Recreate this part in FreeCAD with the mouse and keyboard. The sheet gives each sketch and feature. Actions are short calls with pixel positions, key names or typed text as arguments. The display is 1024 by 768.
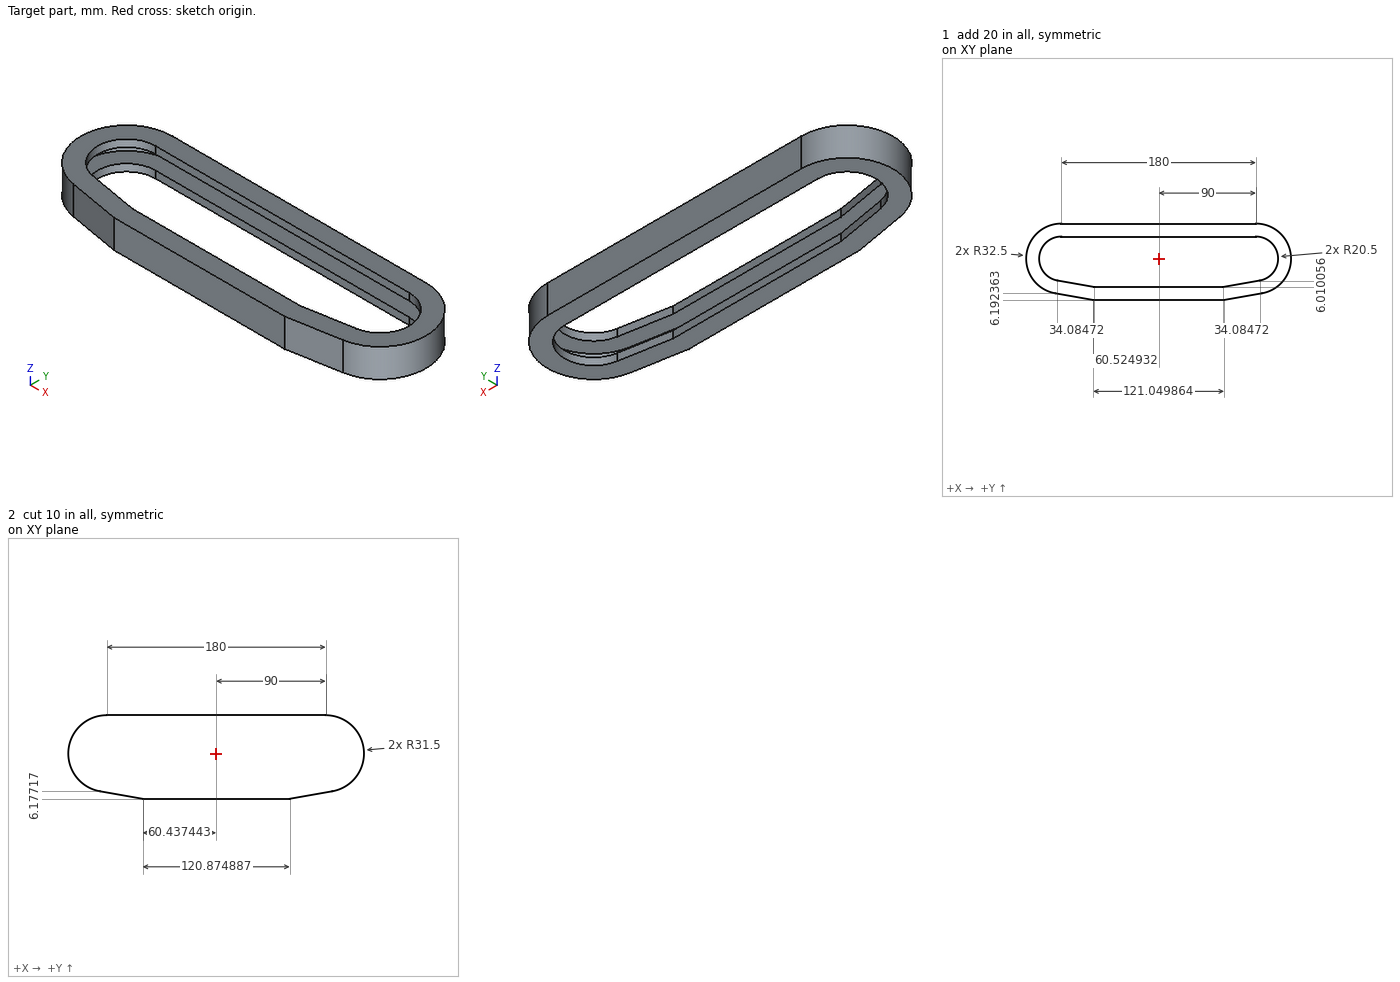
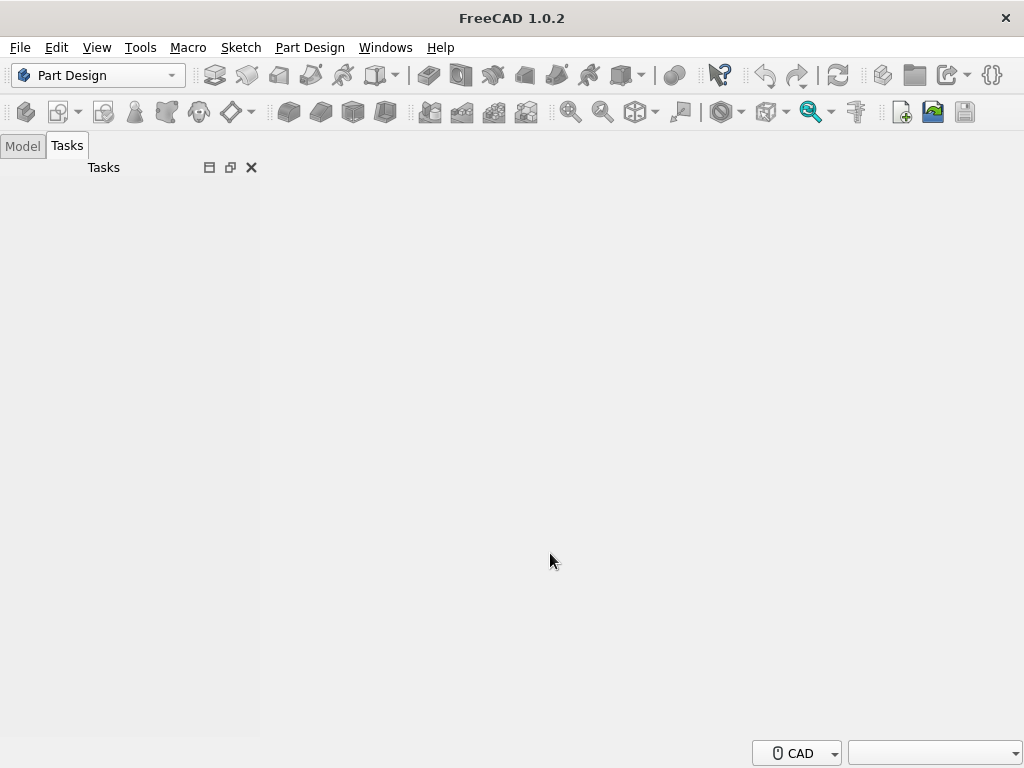
key(ctrl+n)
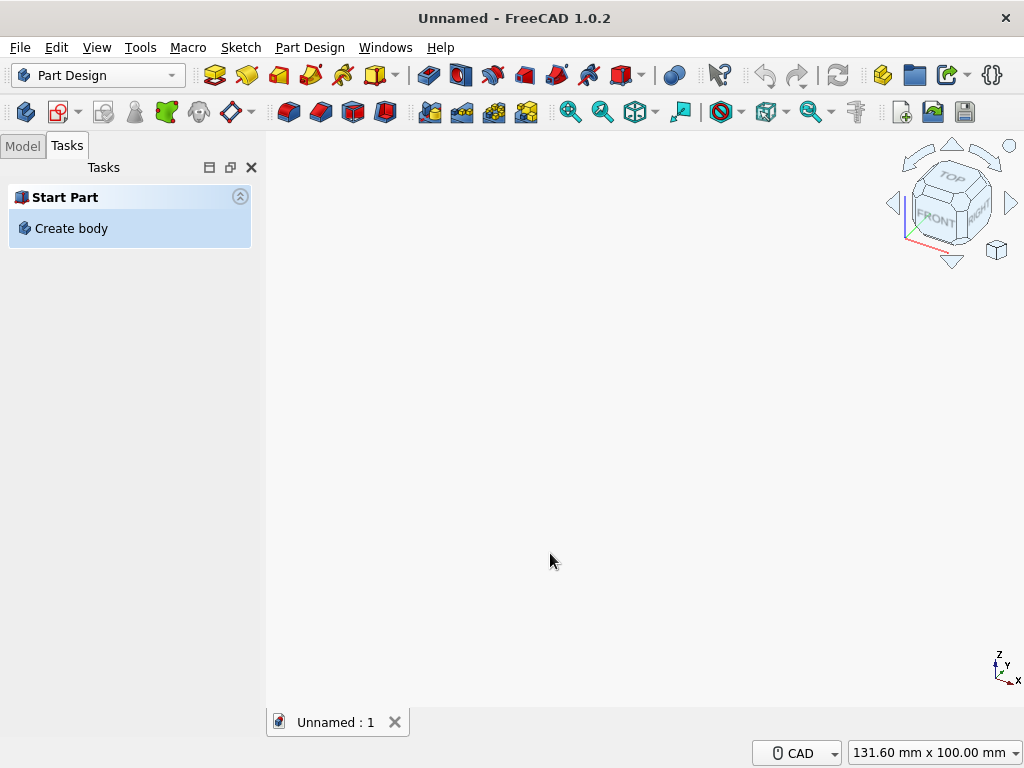
click(58, 112)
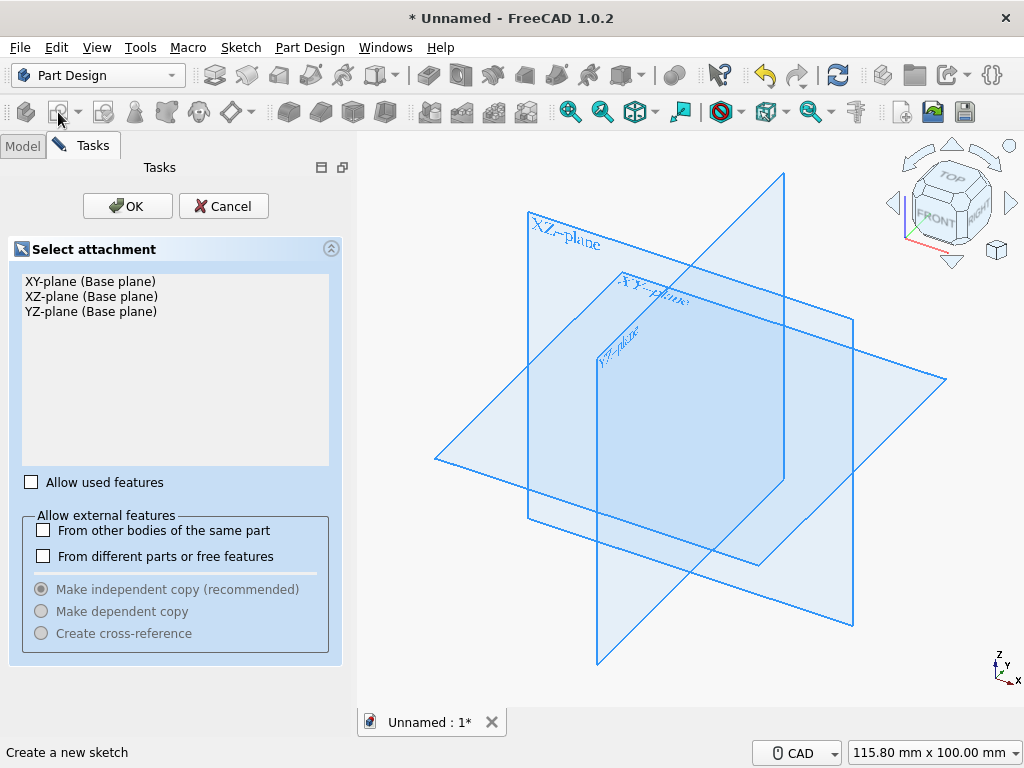
click(82, 282)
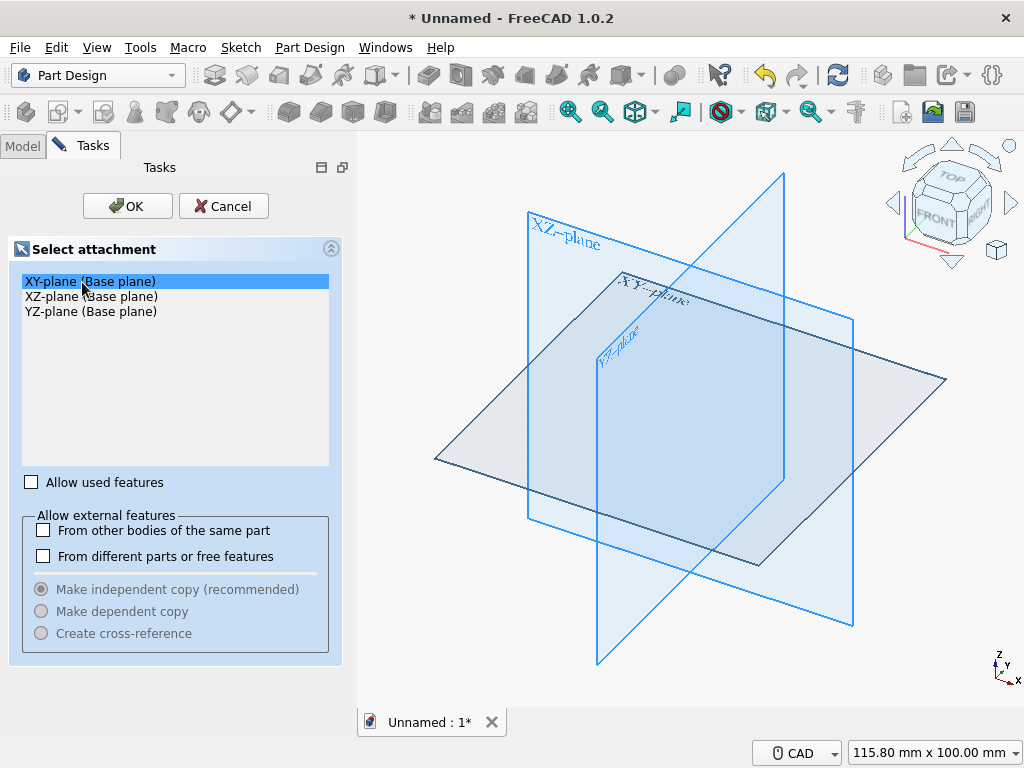
click(128, 206)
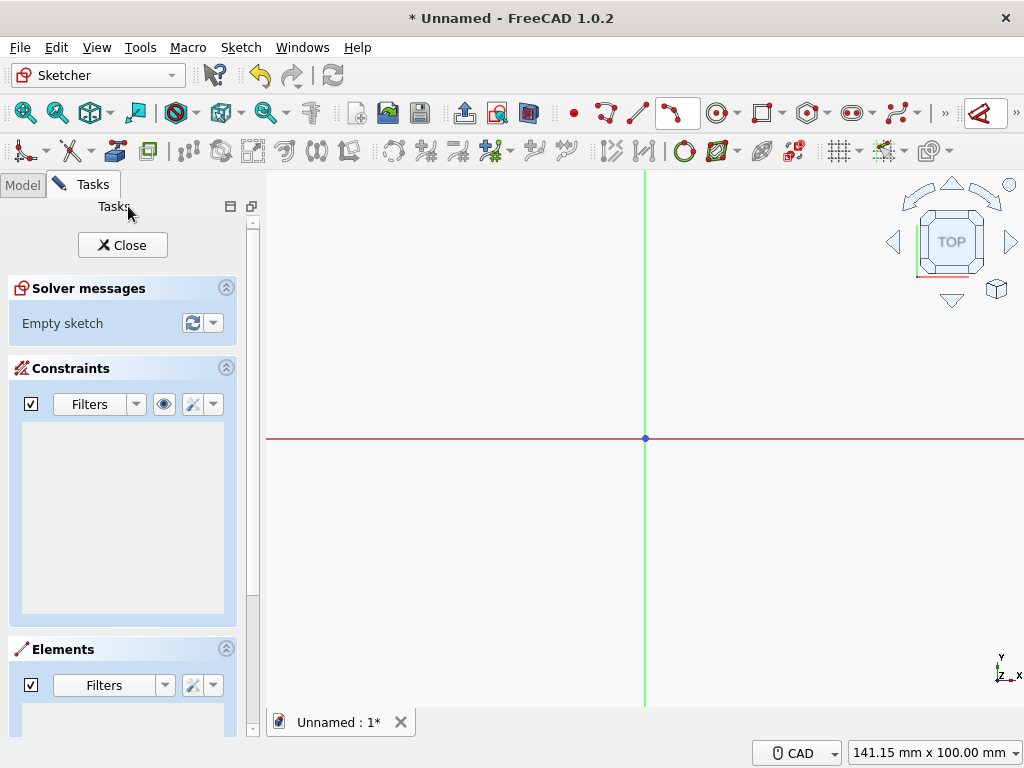
scroll(547, 432, down, 6)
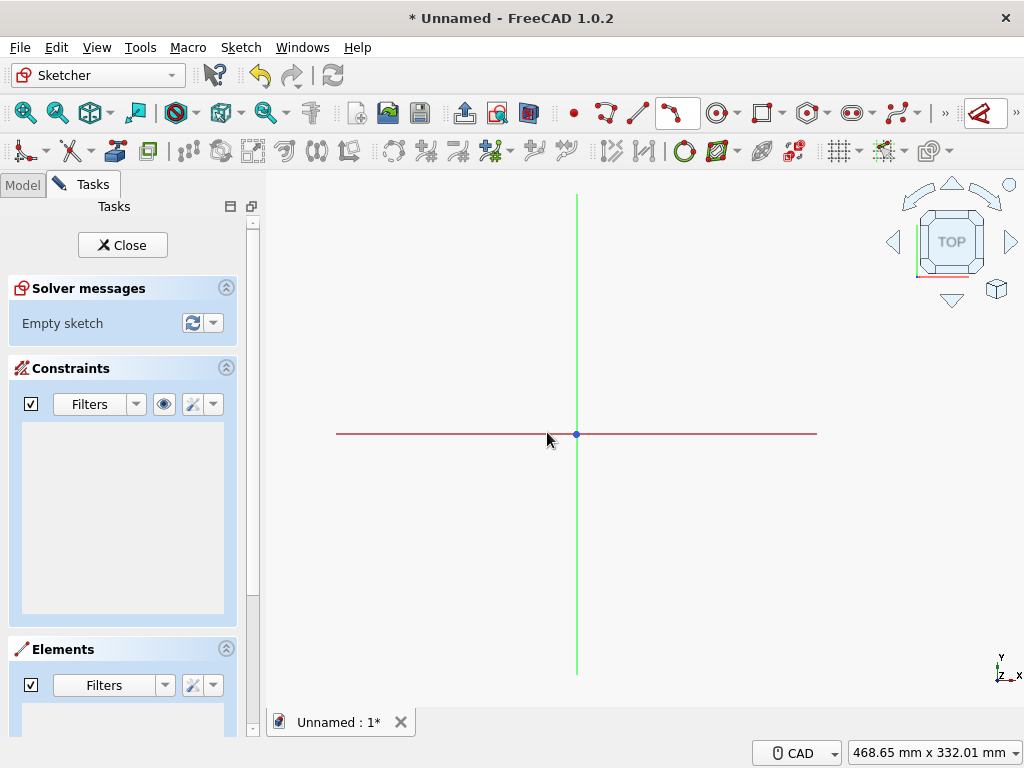
click(638, 114)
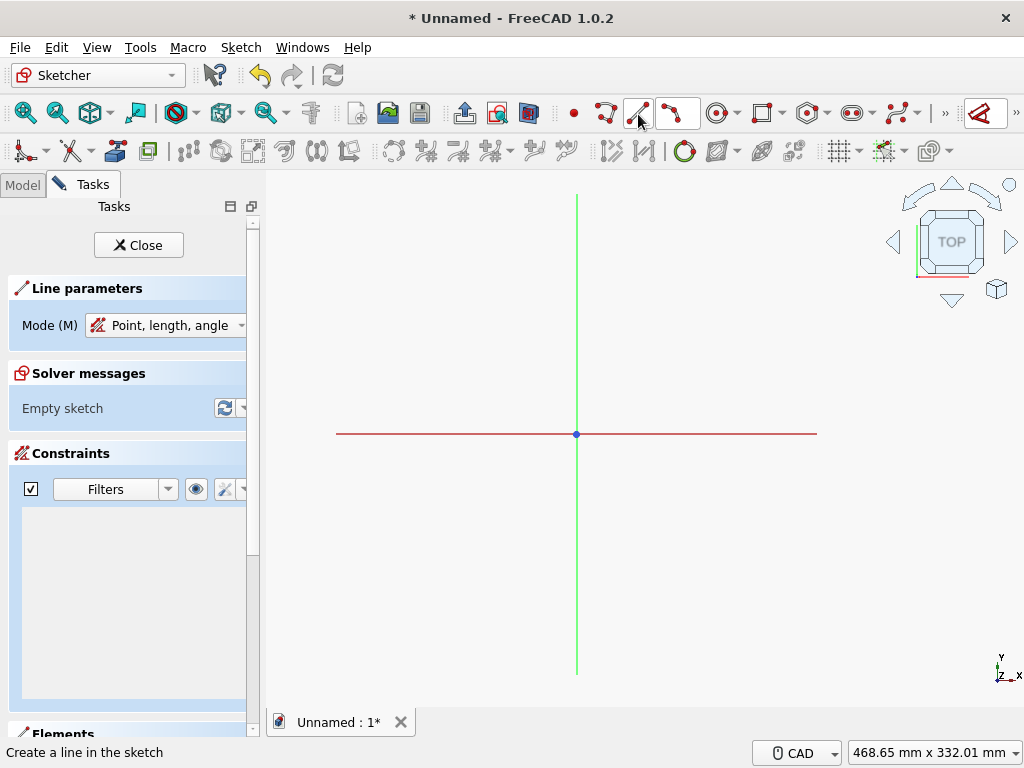
click(722, 382)
click(431, 382)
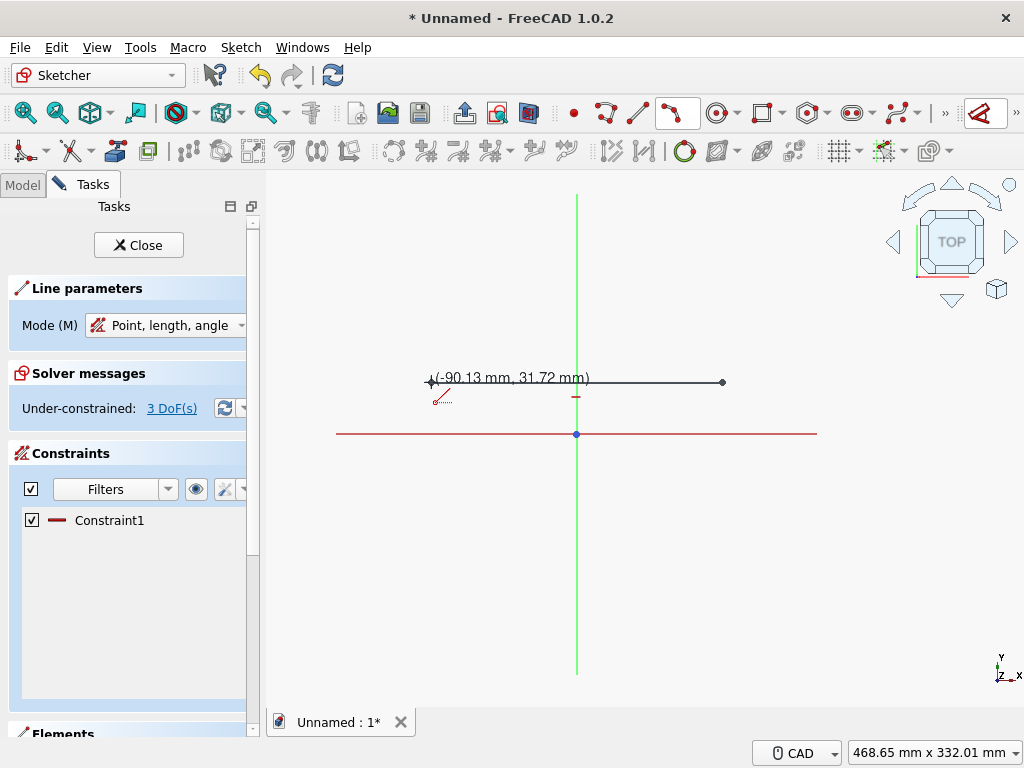
click(606, 114)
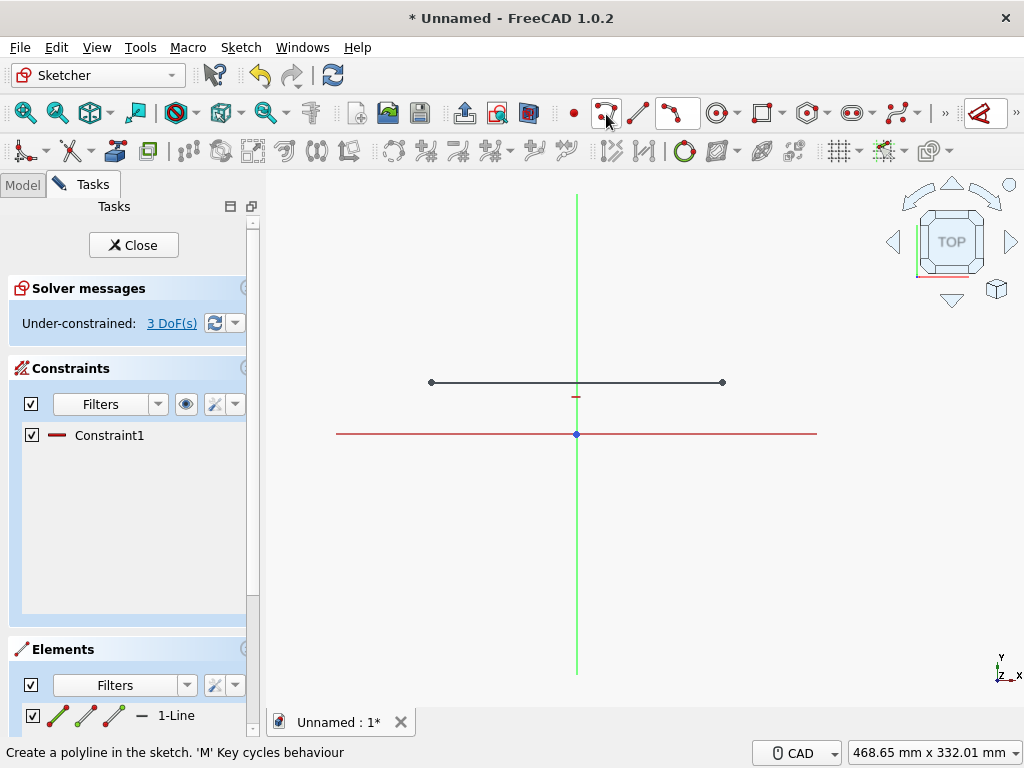
click(422, 486)
click(479, 496)
click(675, 496)
click(731, 486)
right_click(731, 486)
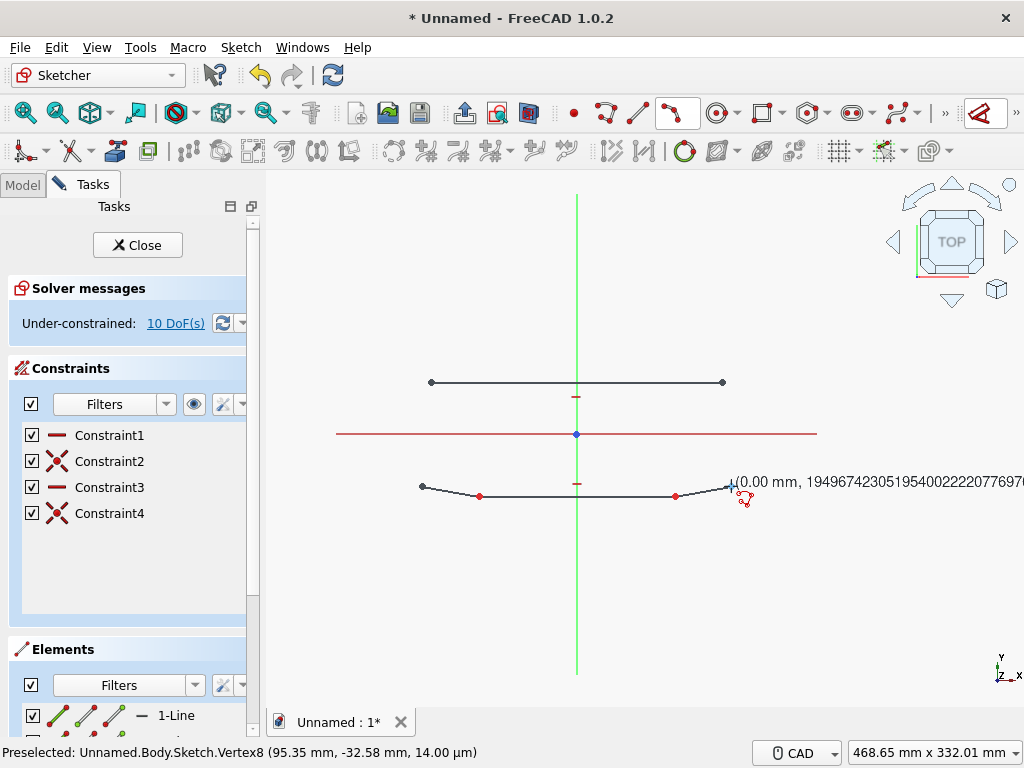
click(672, 114)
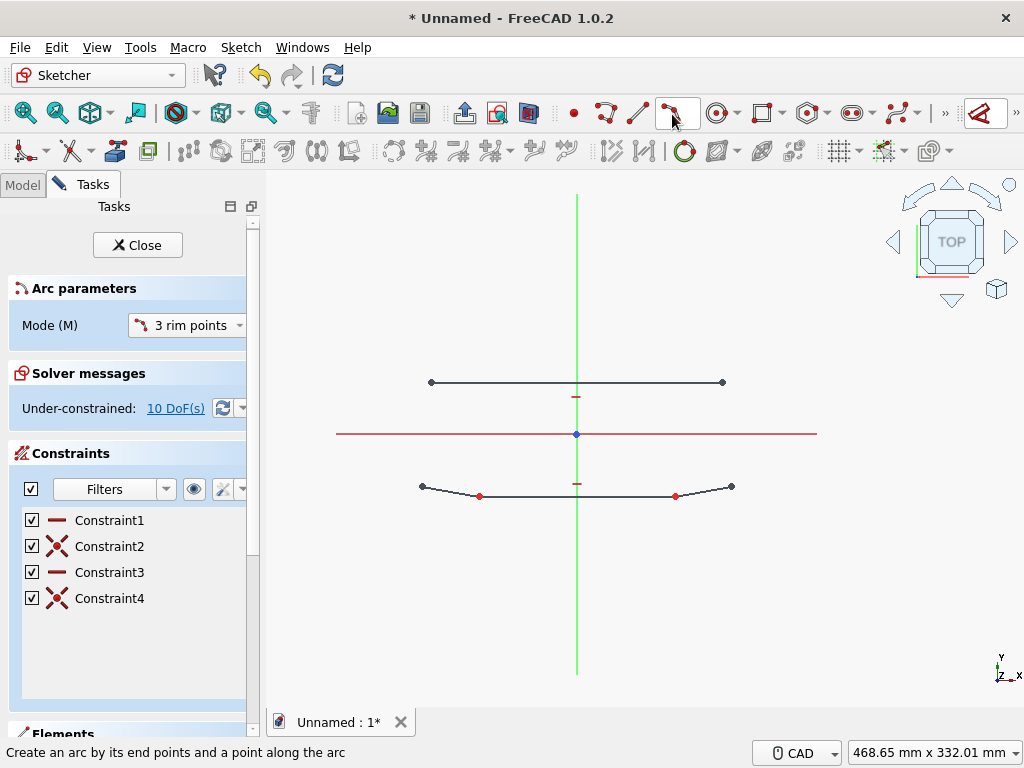
click(431, 383)
click(422, 487)
click(382, 415)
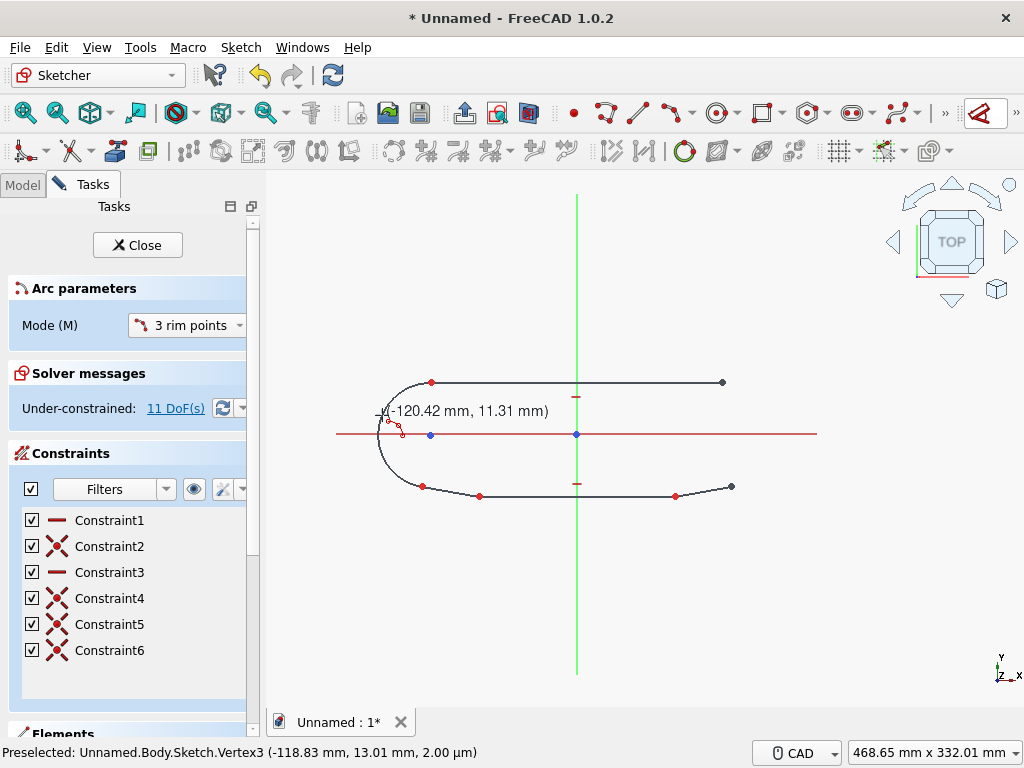
click(731, 487)
click(722, 383)
click(771, 415)